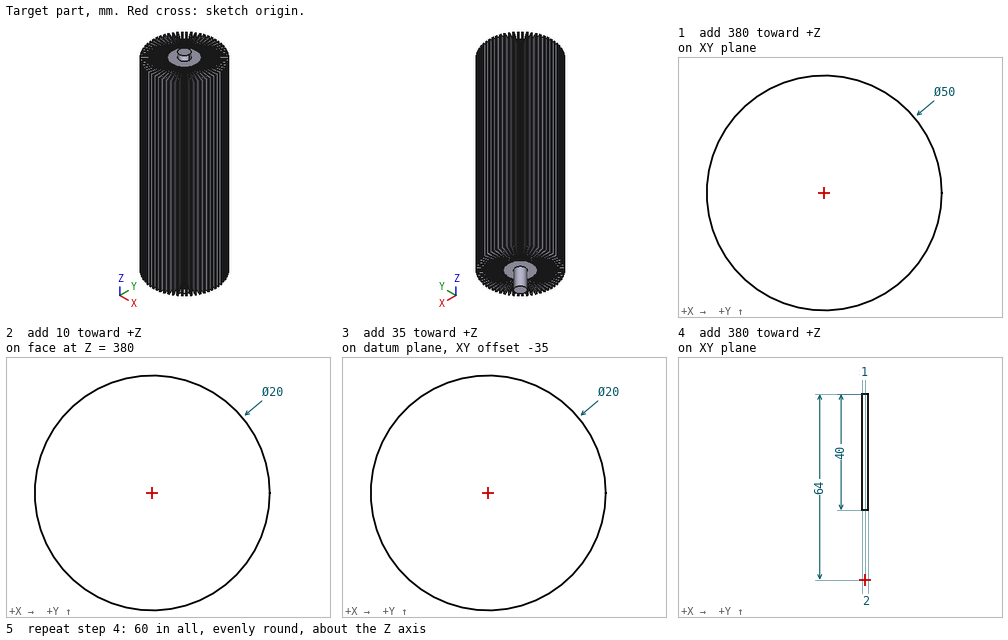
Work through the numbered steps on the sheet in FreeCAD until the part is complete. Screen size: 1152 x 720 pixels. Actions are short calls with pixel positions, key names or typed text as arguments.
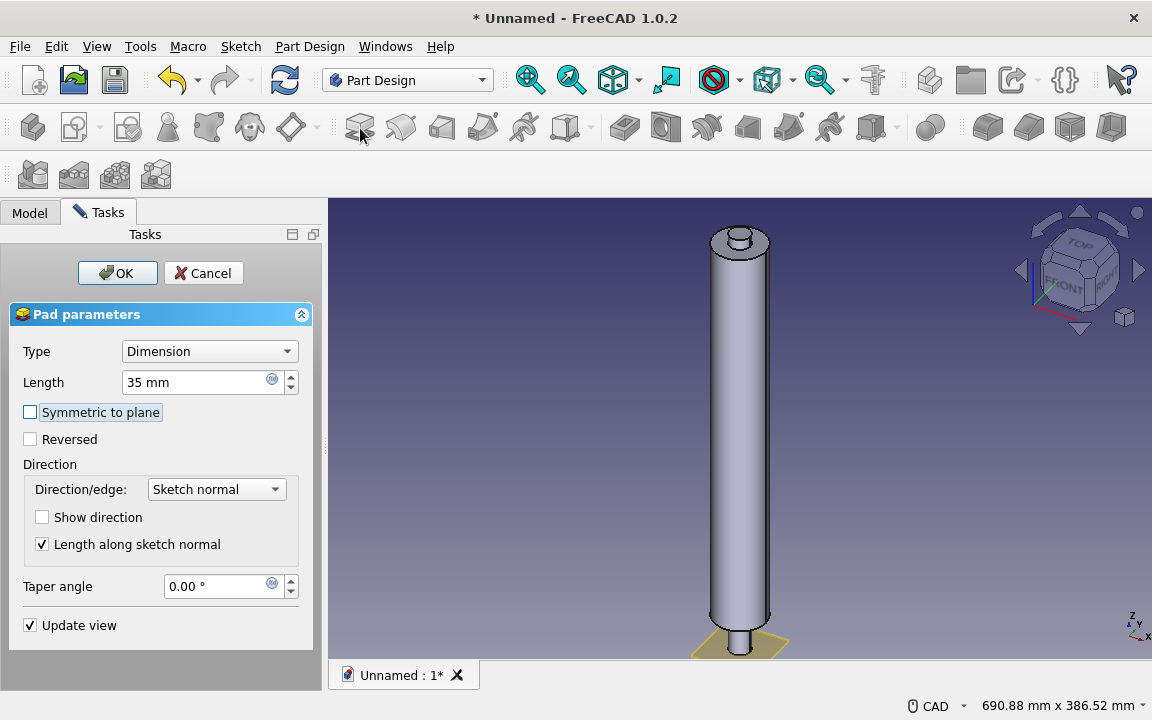
click(118, 273)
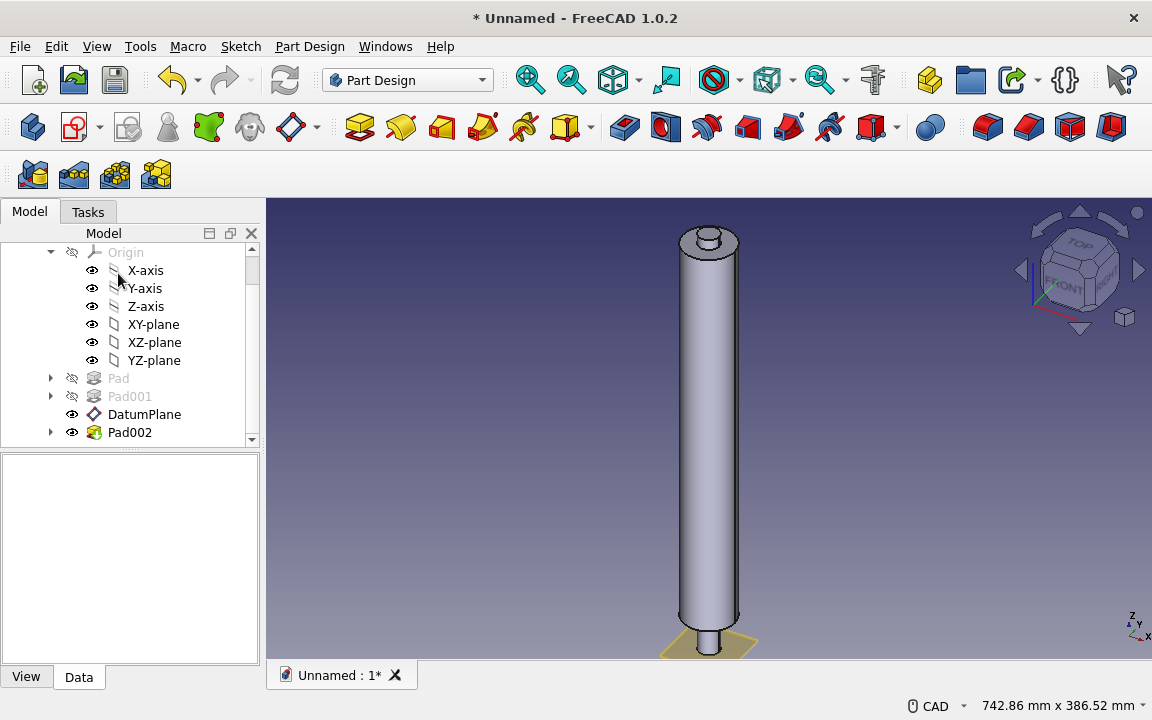
click(117, 414)
key(space)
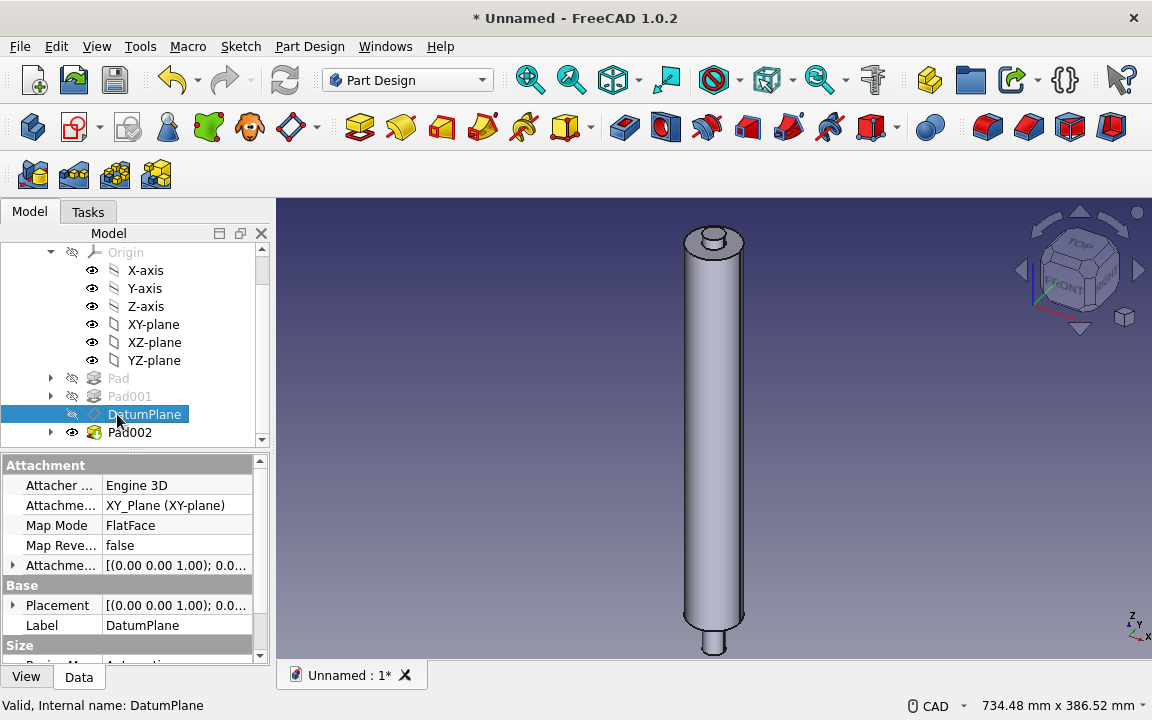
click(531, 80)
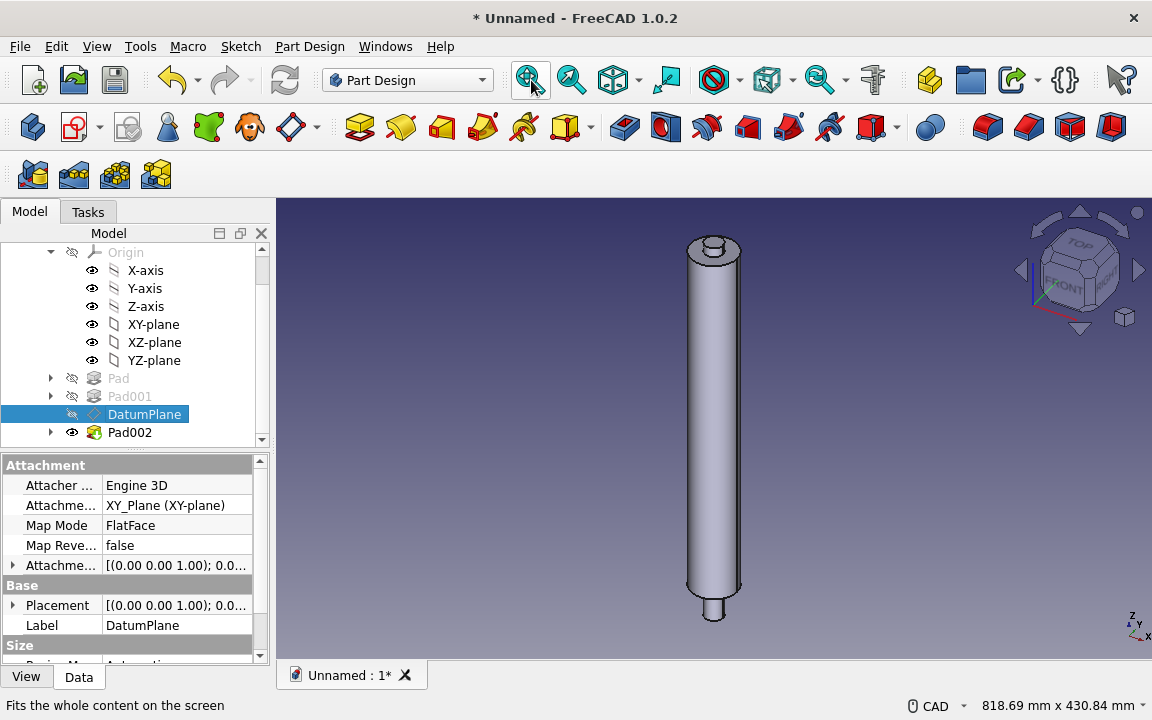
click(316, 619)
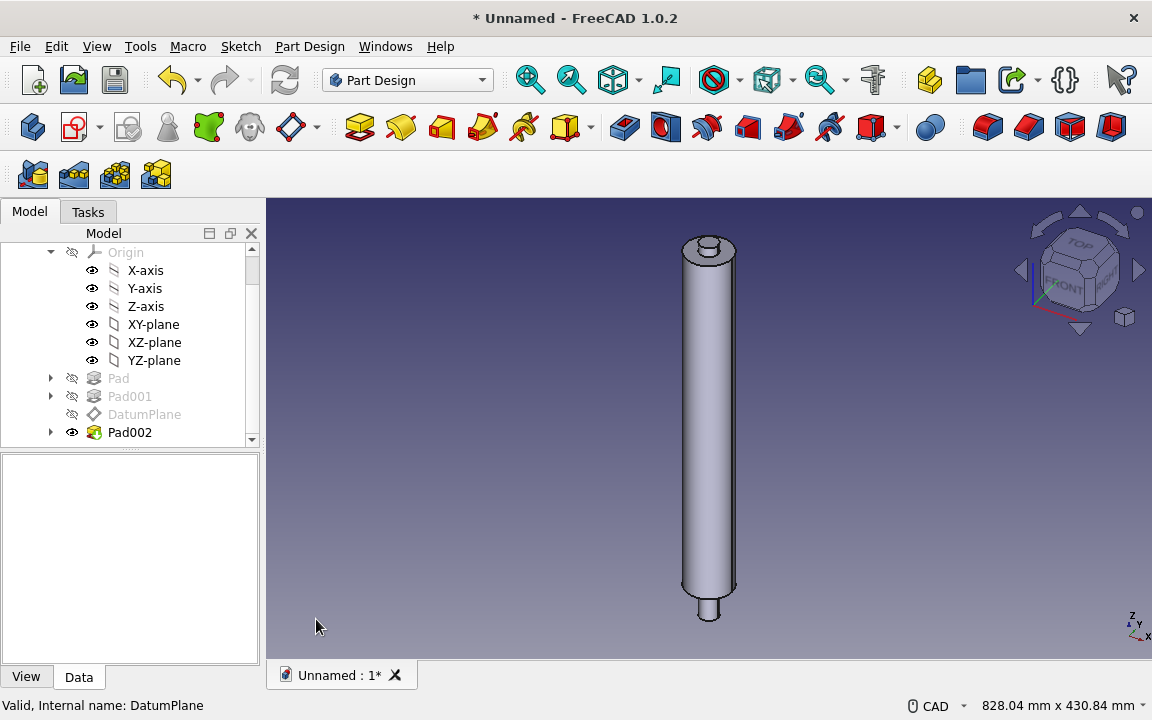
click(74, 128)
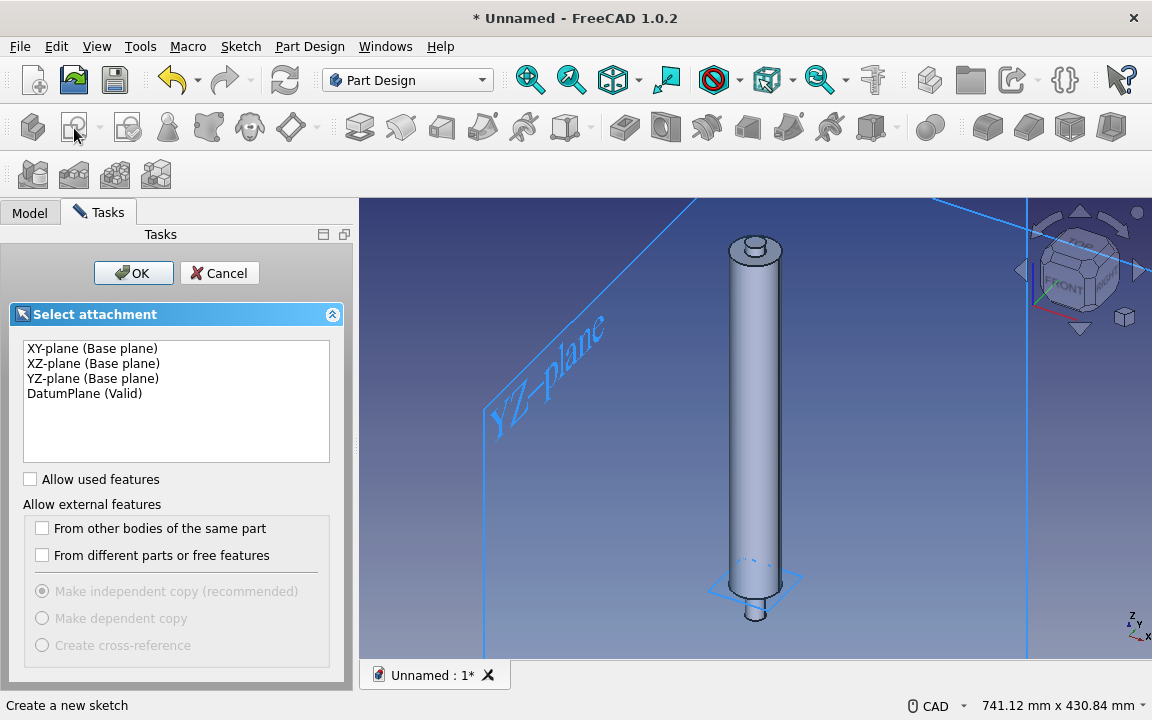
click(84, 348)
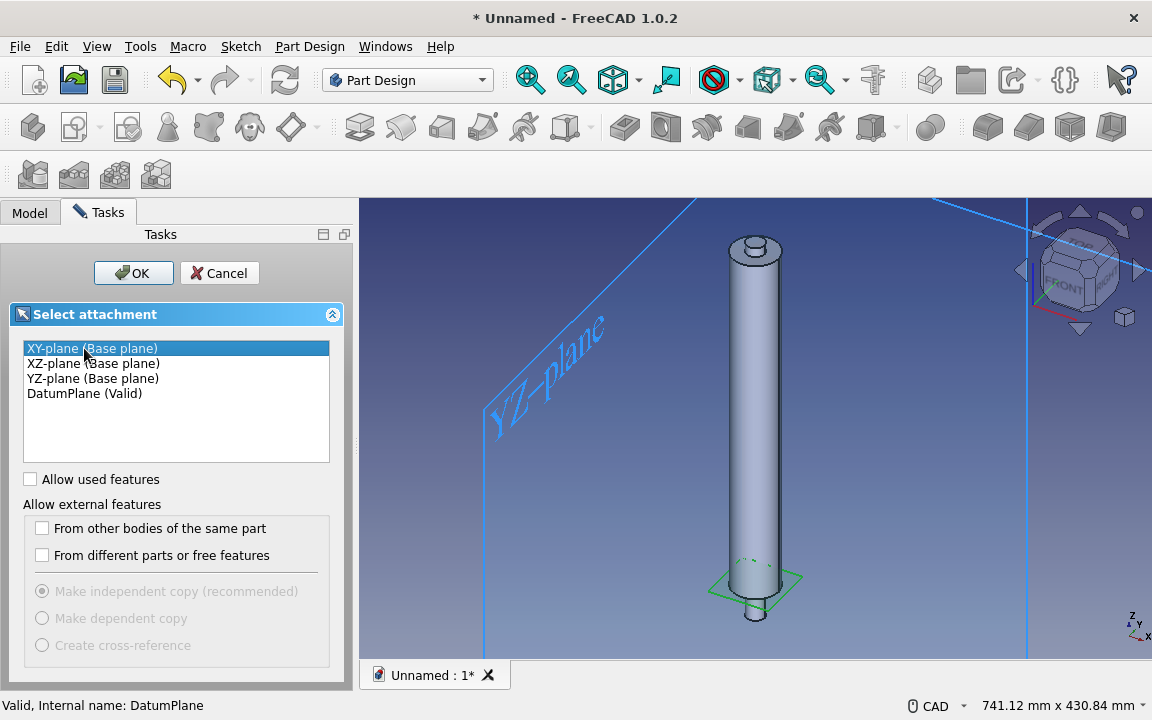
click(134, 273)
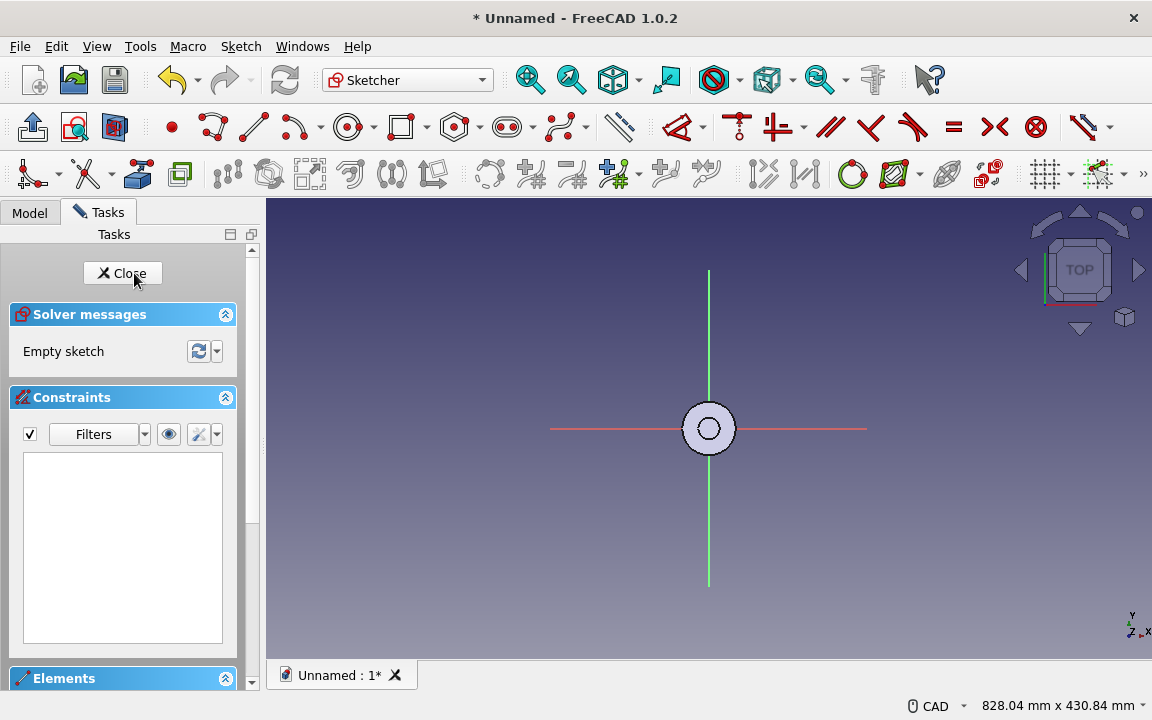
click(115, 128)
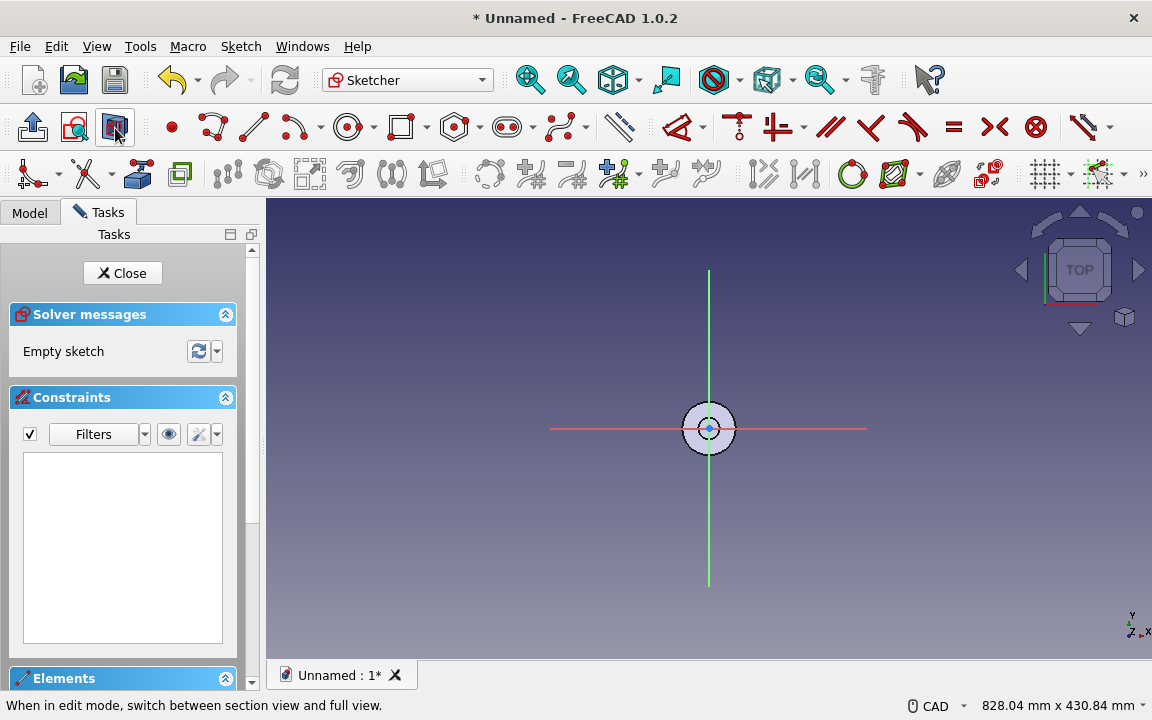
scroll(731, 383, up, 7)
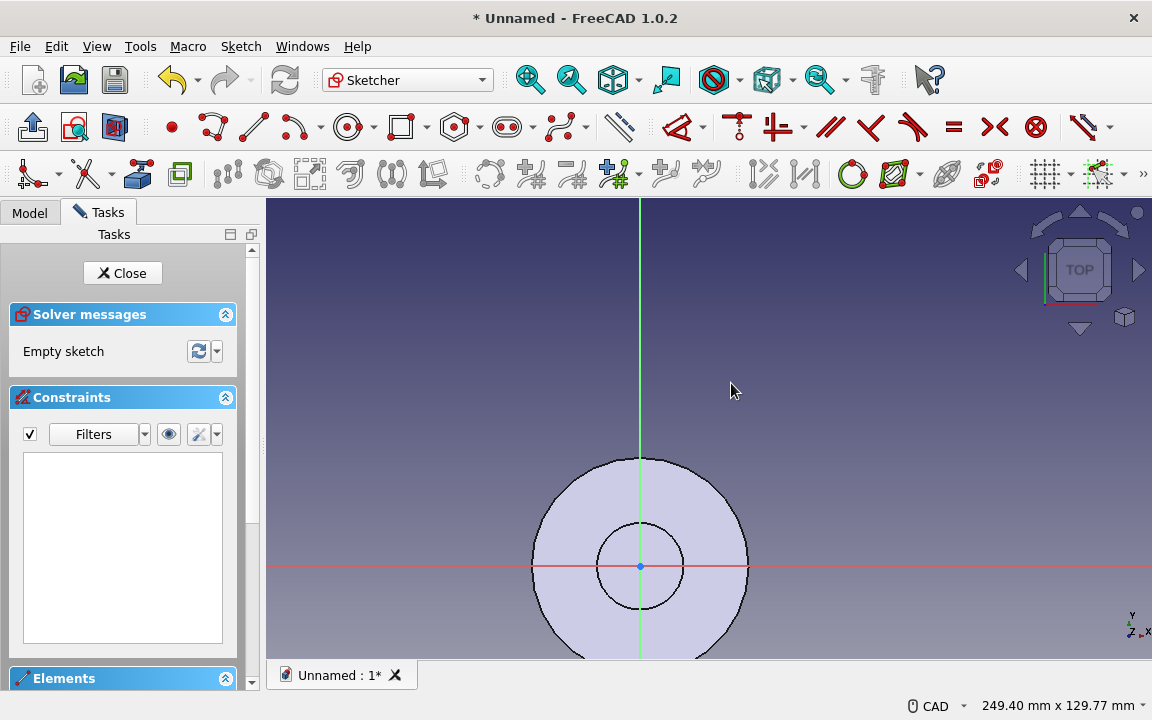
click(400, 128)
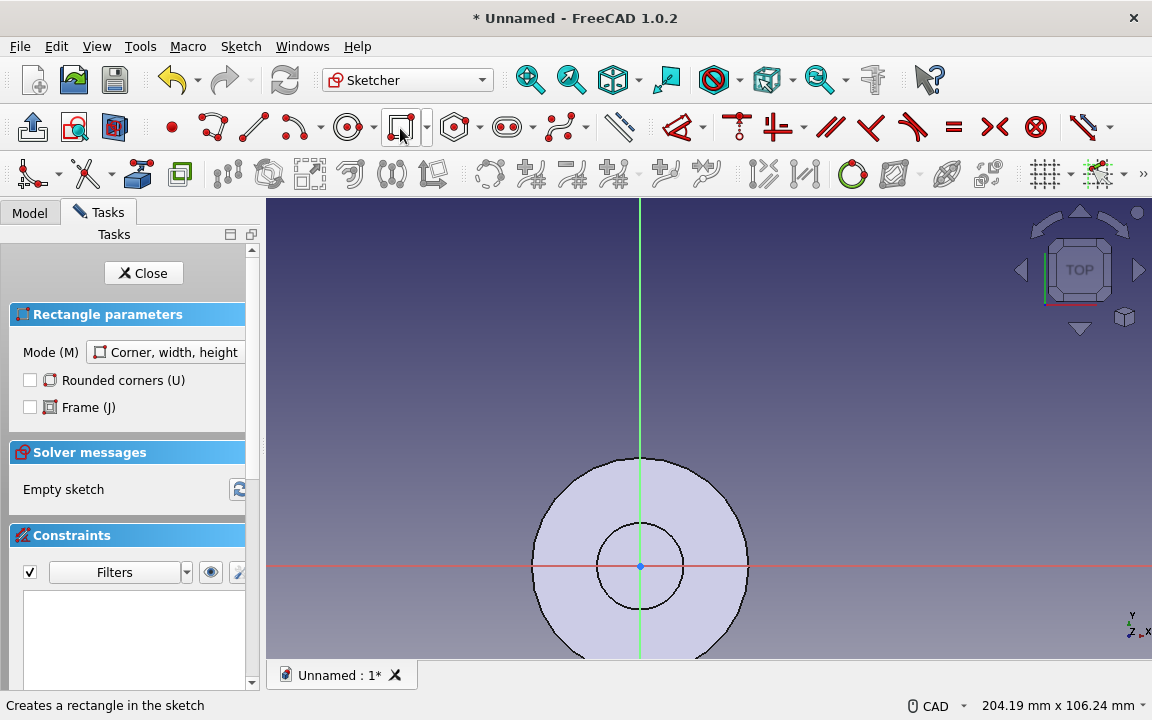
scroll(636, 289, up, 7)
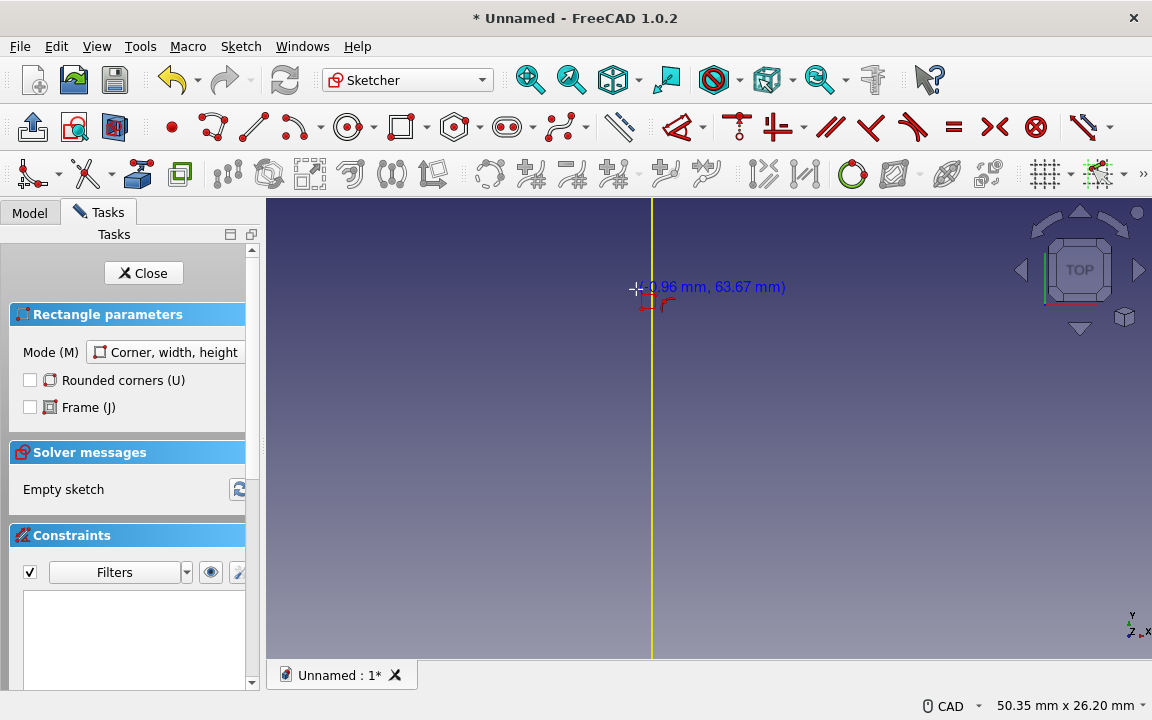
click(634, 287)